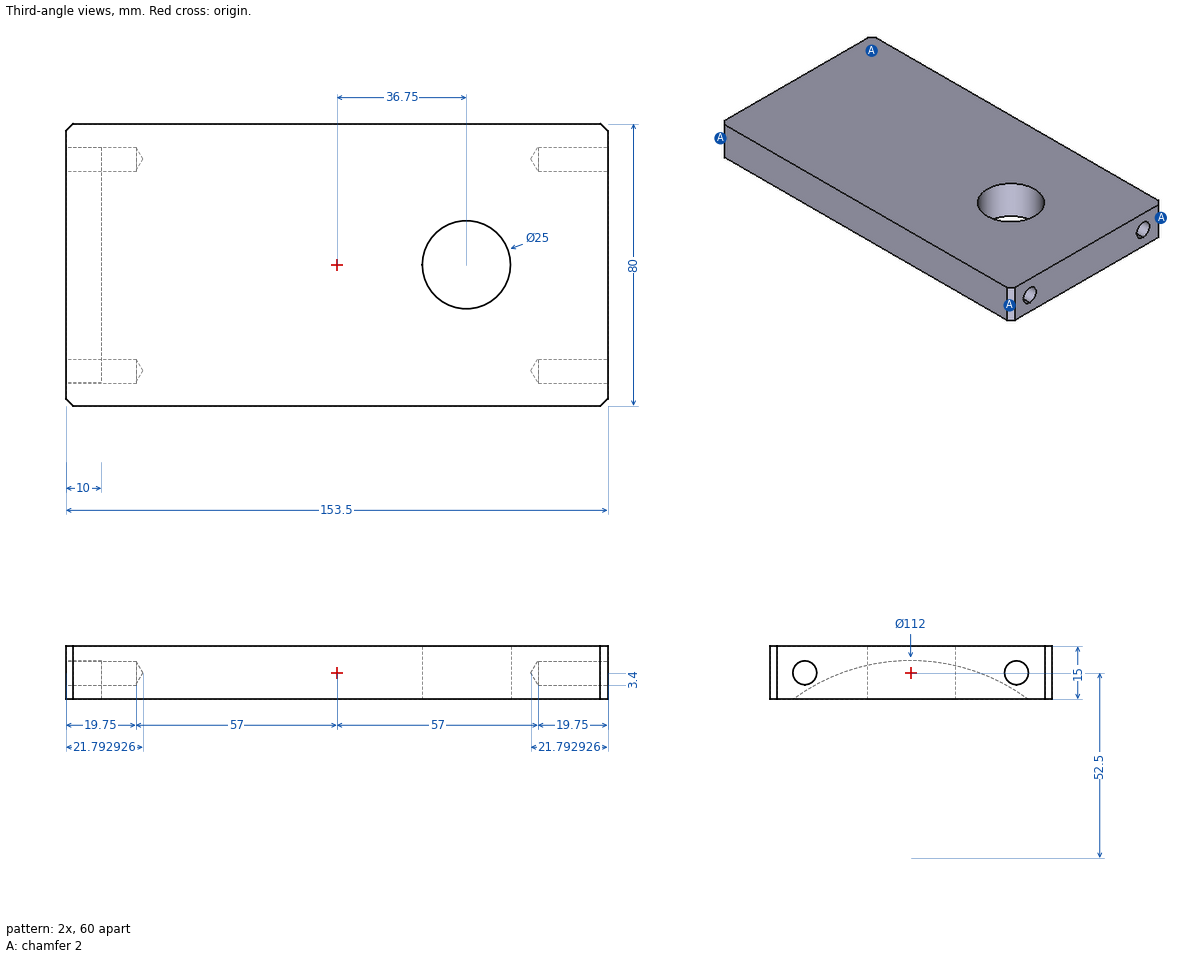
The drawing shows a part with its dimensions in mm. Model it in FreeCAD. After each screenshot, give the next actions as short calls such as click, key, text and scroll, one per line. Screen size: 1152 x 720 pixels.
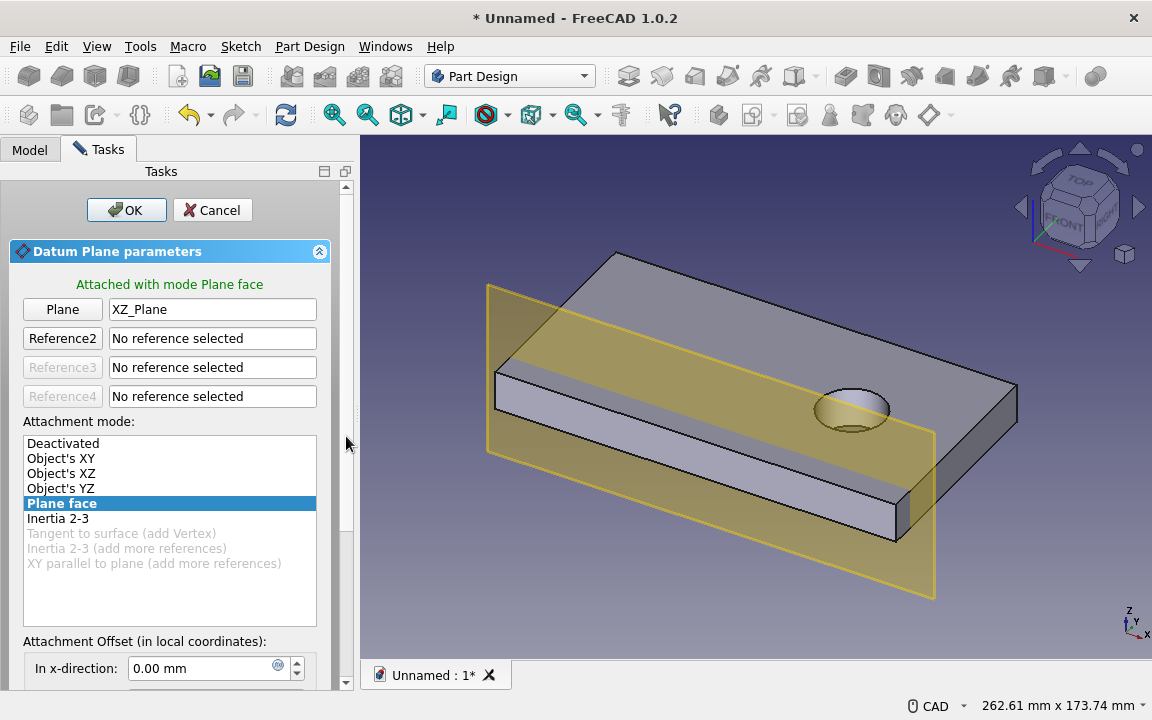
click(127, 210)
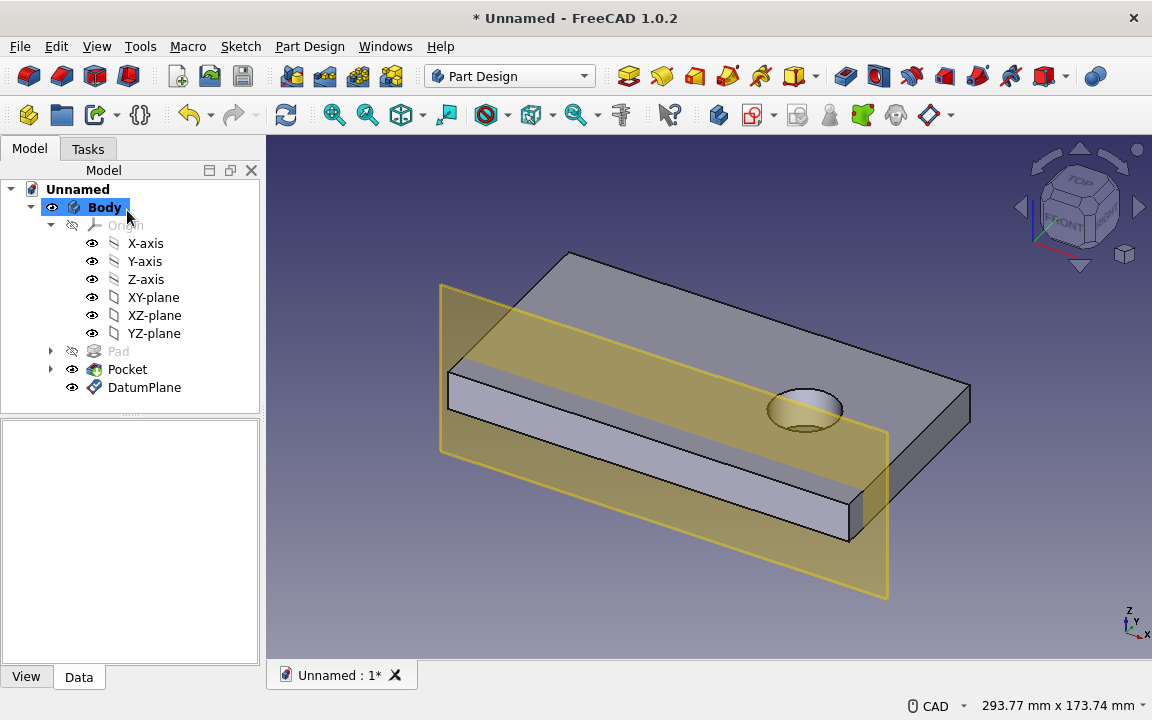
click(117, 387)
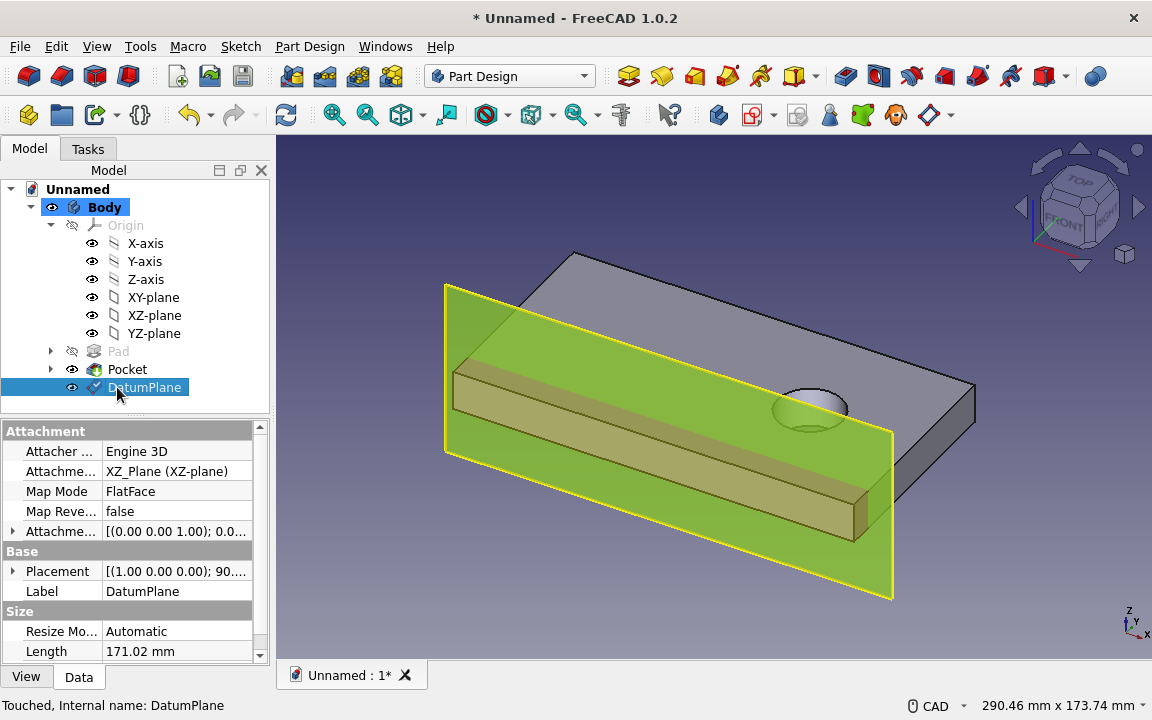
click(752, 116)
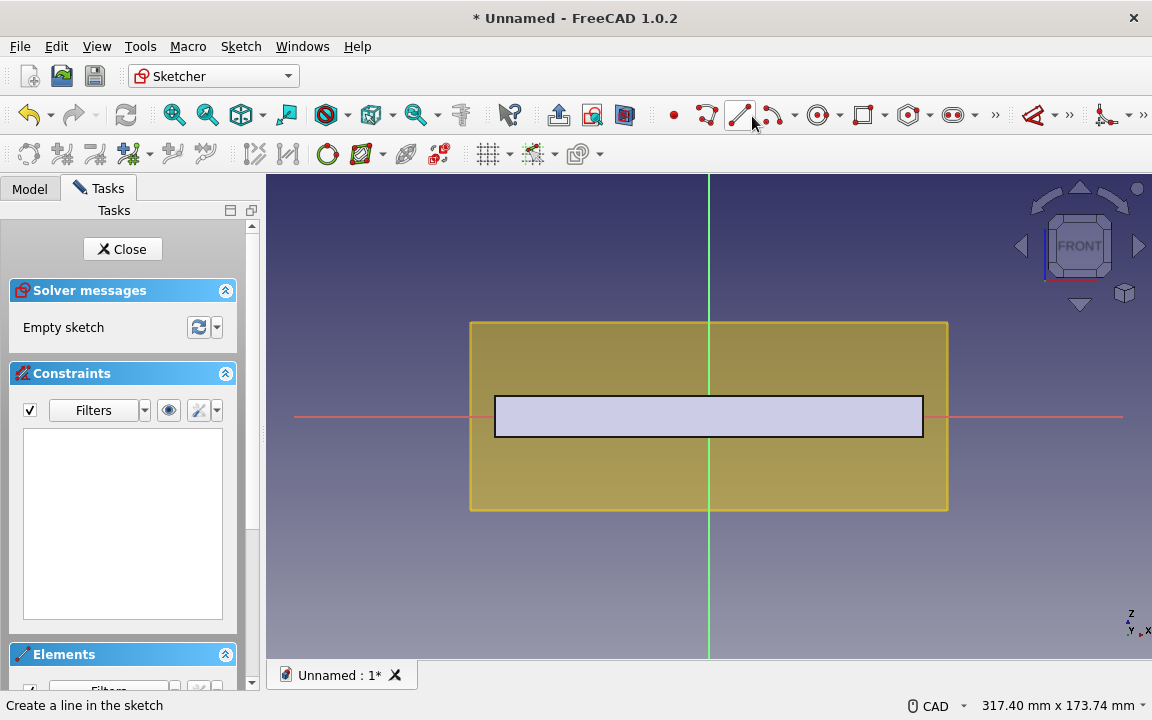
click(625, 116)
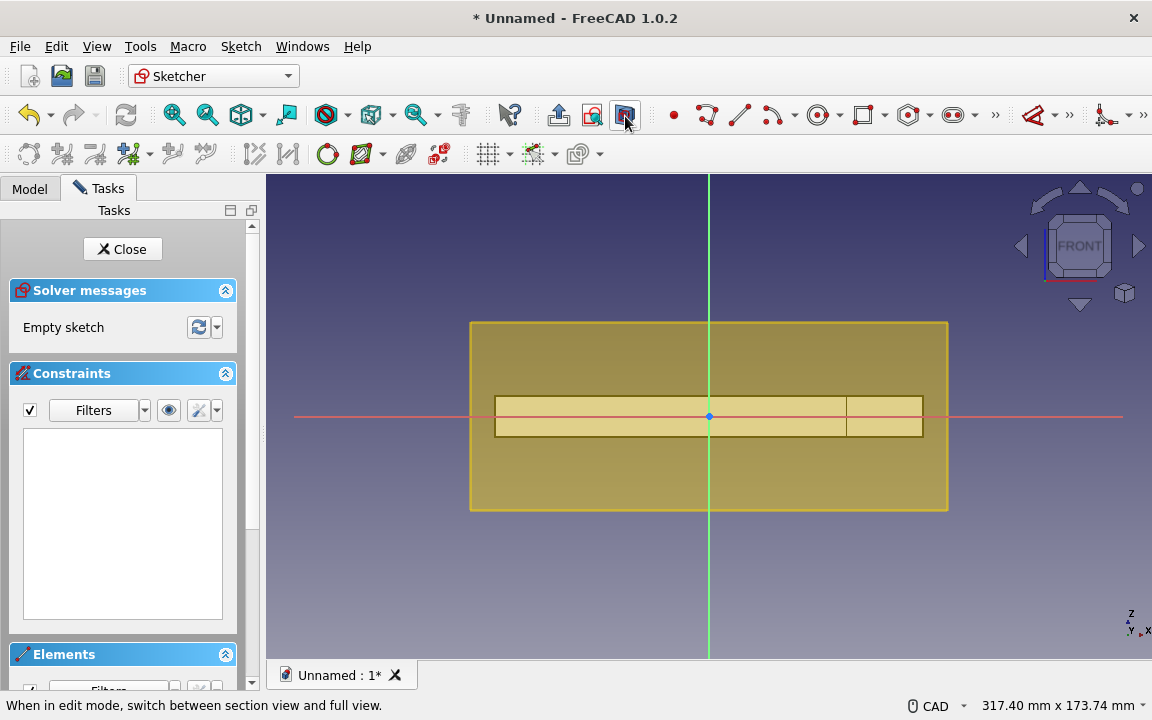
scroll(932, 422, up, 10)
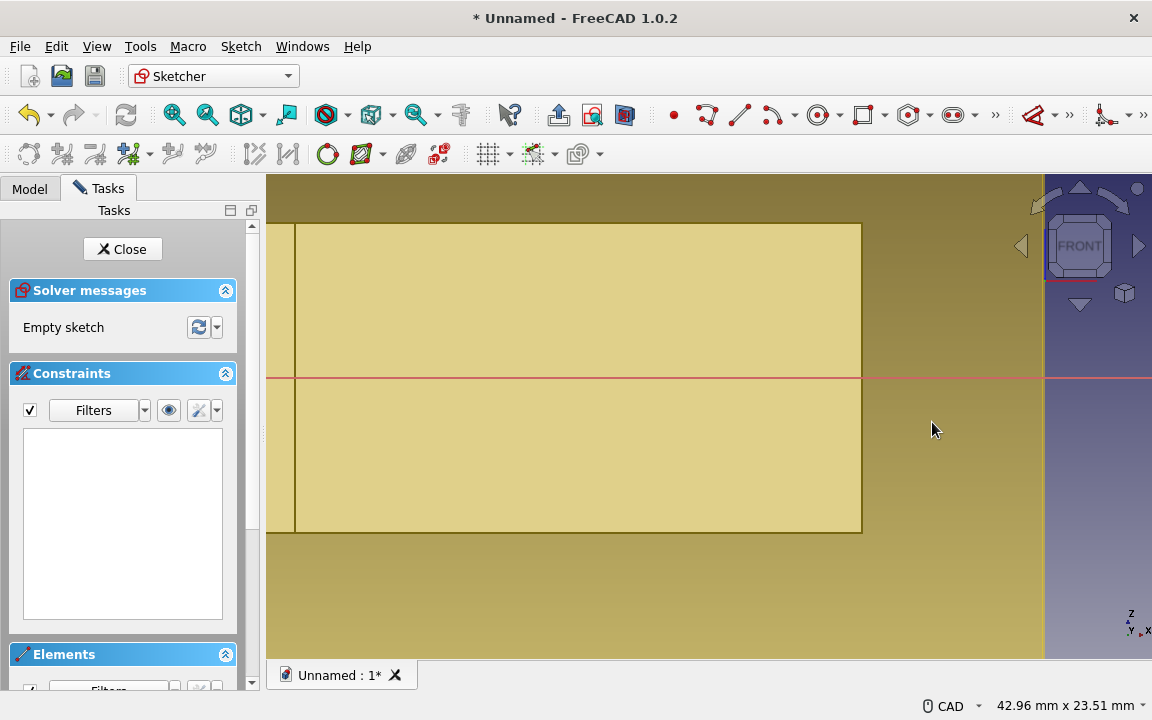
key(g)
key(m)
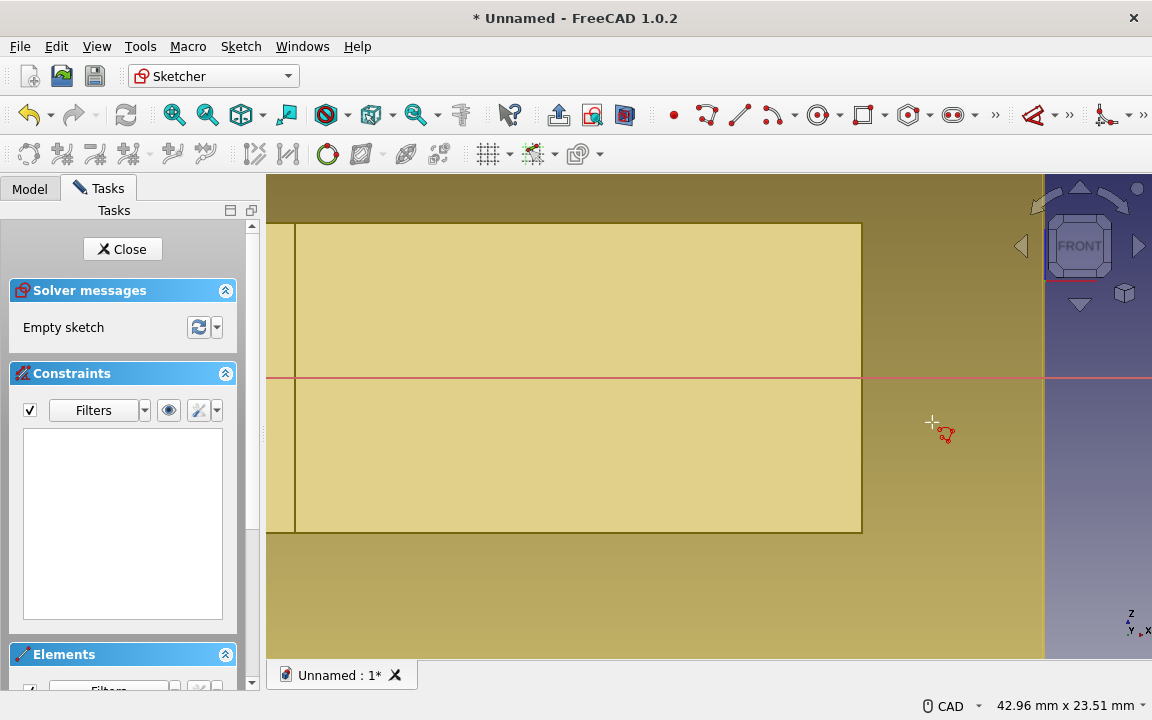
click(413, 378)
click(862, 387)
click(862, 448)
click(455, 448)
click(413, 378)
key(Escape)
key(Escape)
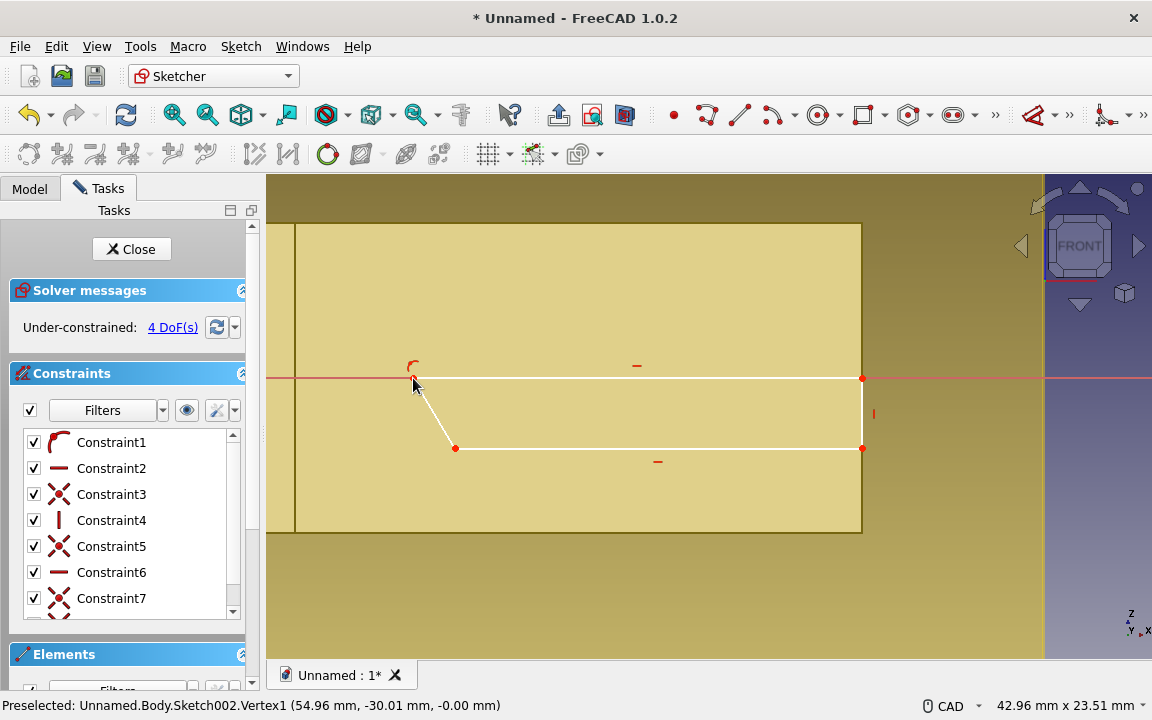
click(1032, 116)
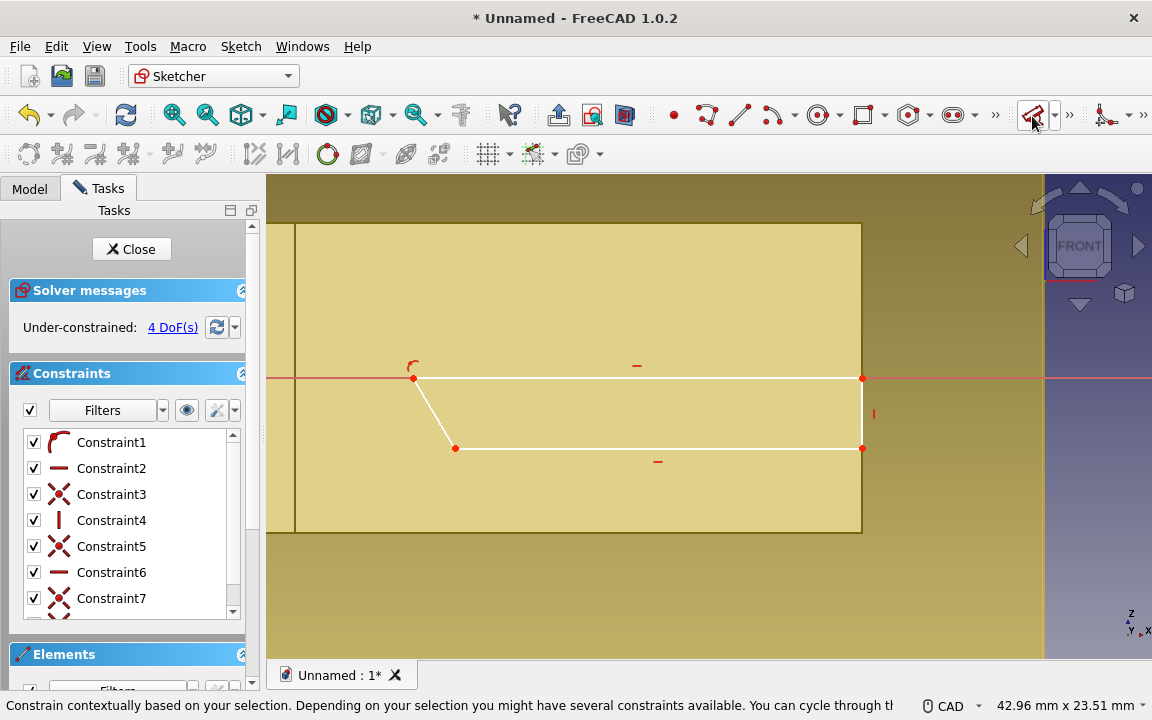
click(862, 399)
click(896, 414)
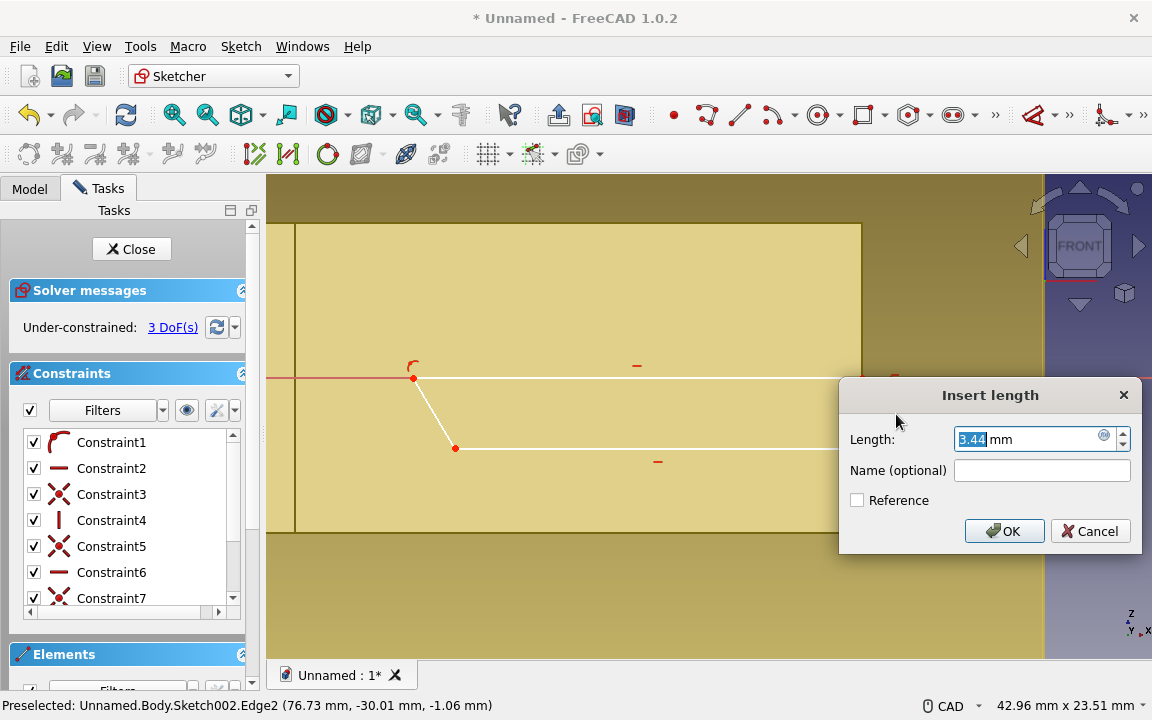
text(3.4)
key(Return)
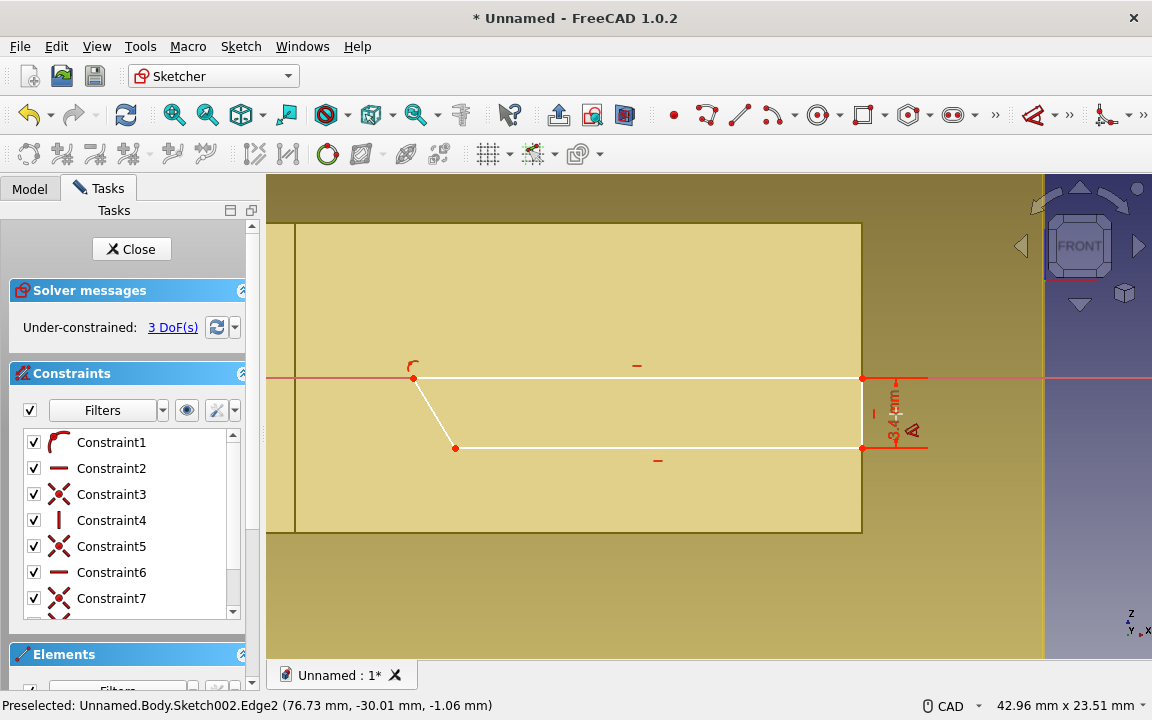
click(455, 448)
click(375, 482)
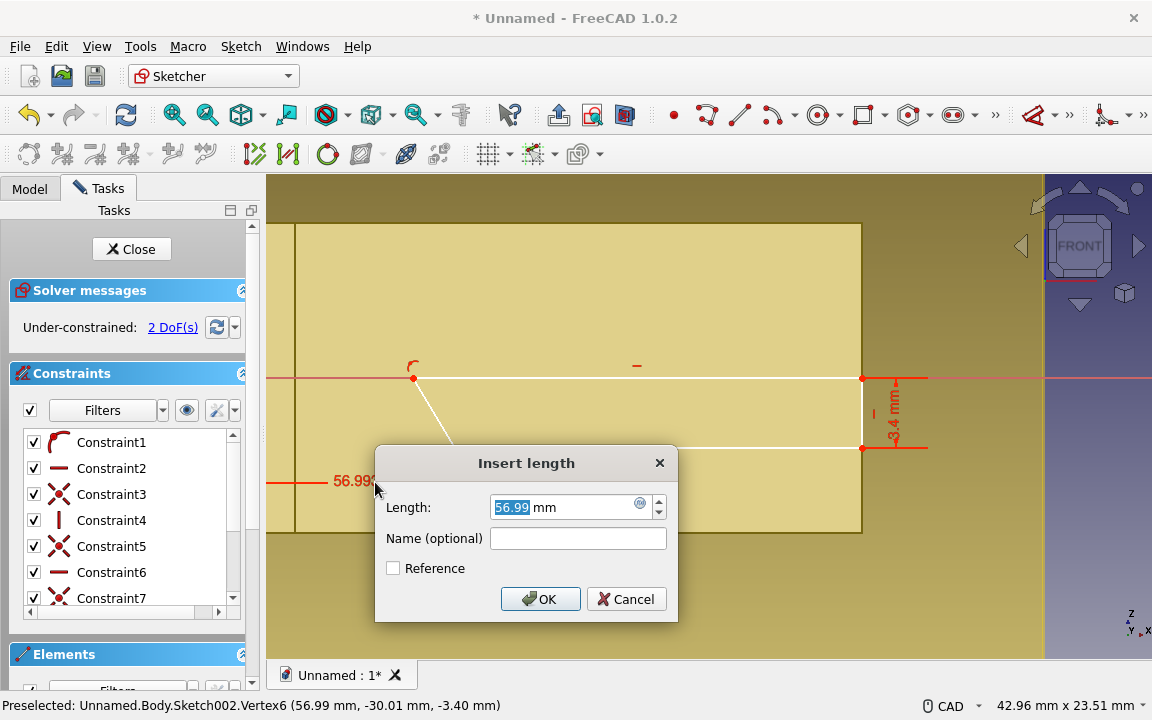
text(57)
key(Return)